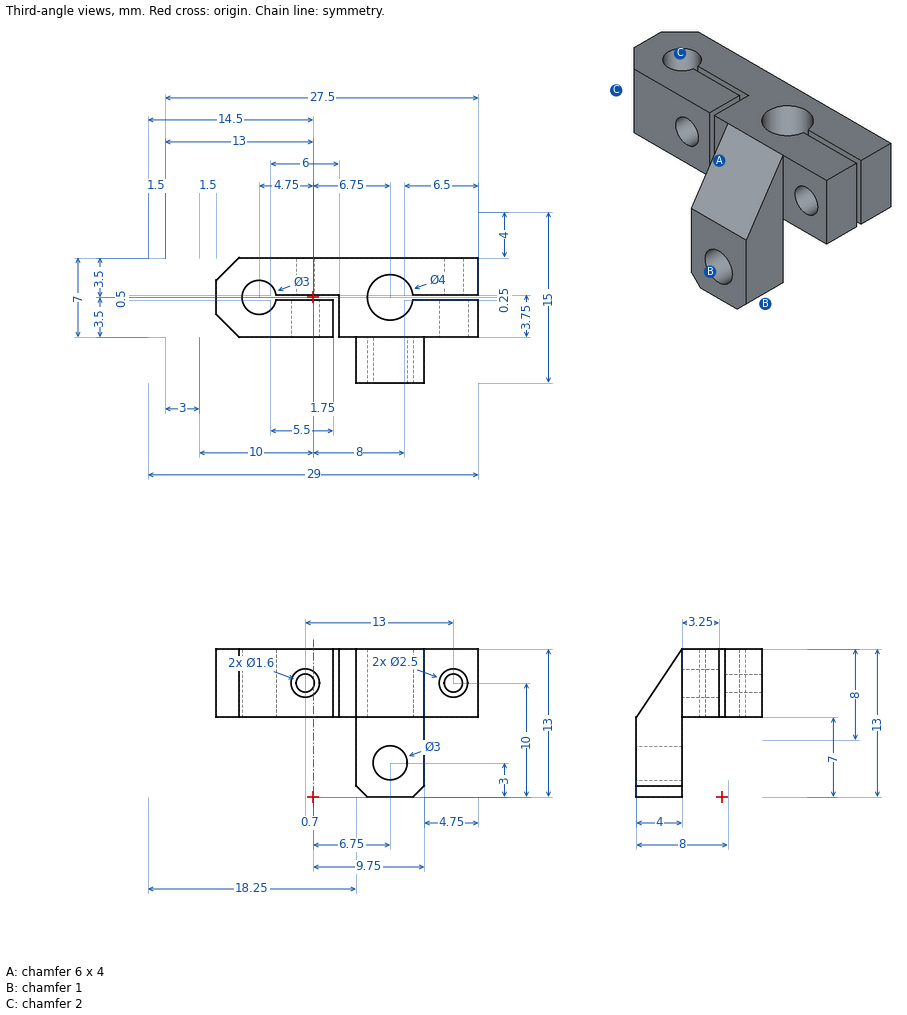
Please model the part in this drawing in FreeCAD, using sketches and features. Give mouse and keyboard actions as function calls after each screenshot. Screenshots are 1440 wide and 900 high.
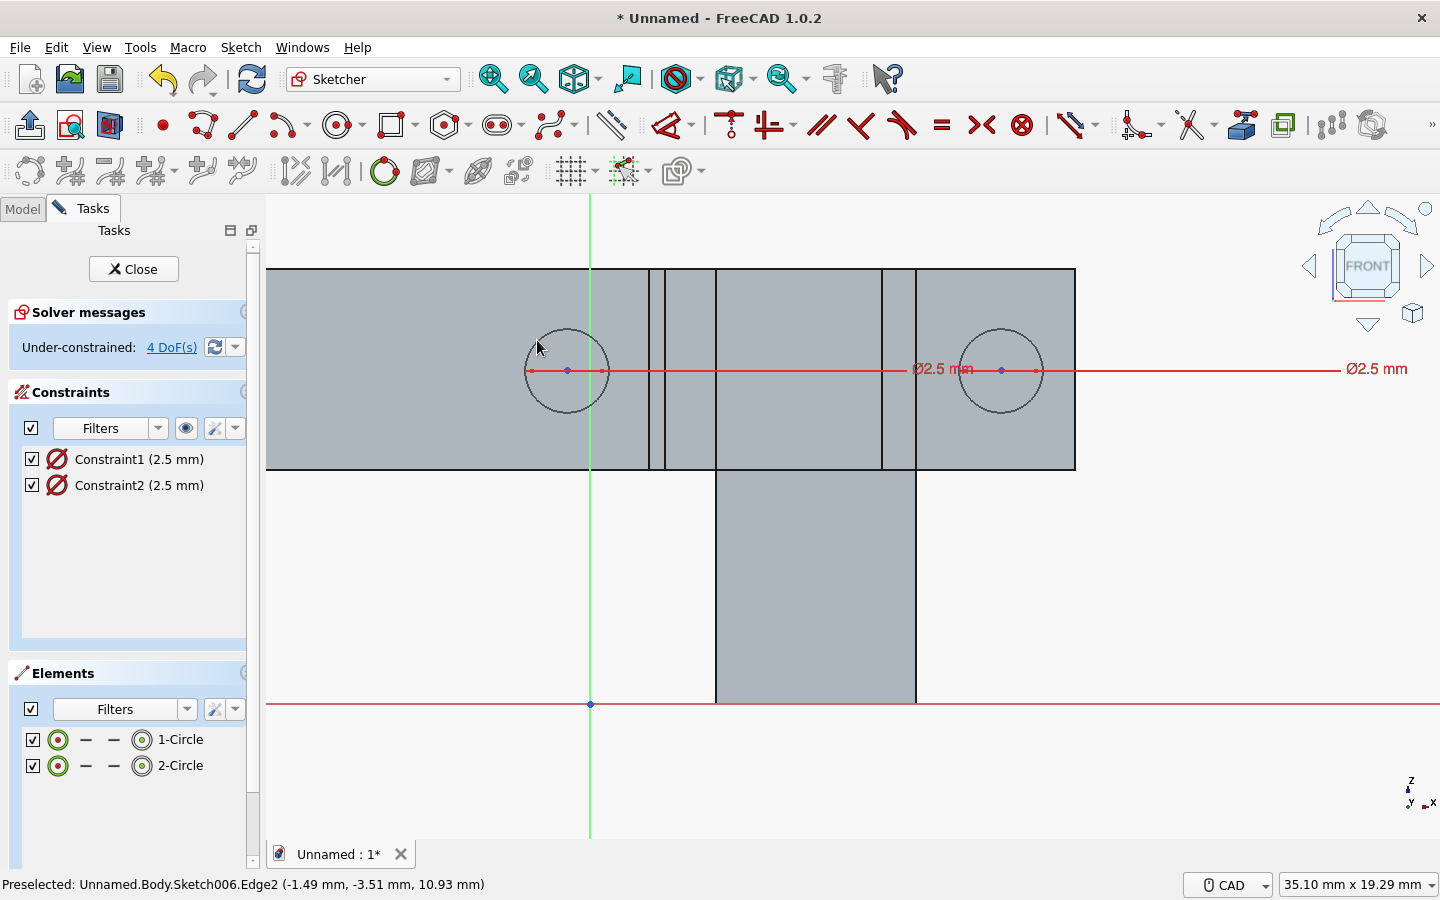
click(1001, 371)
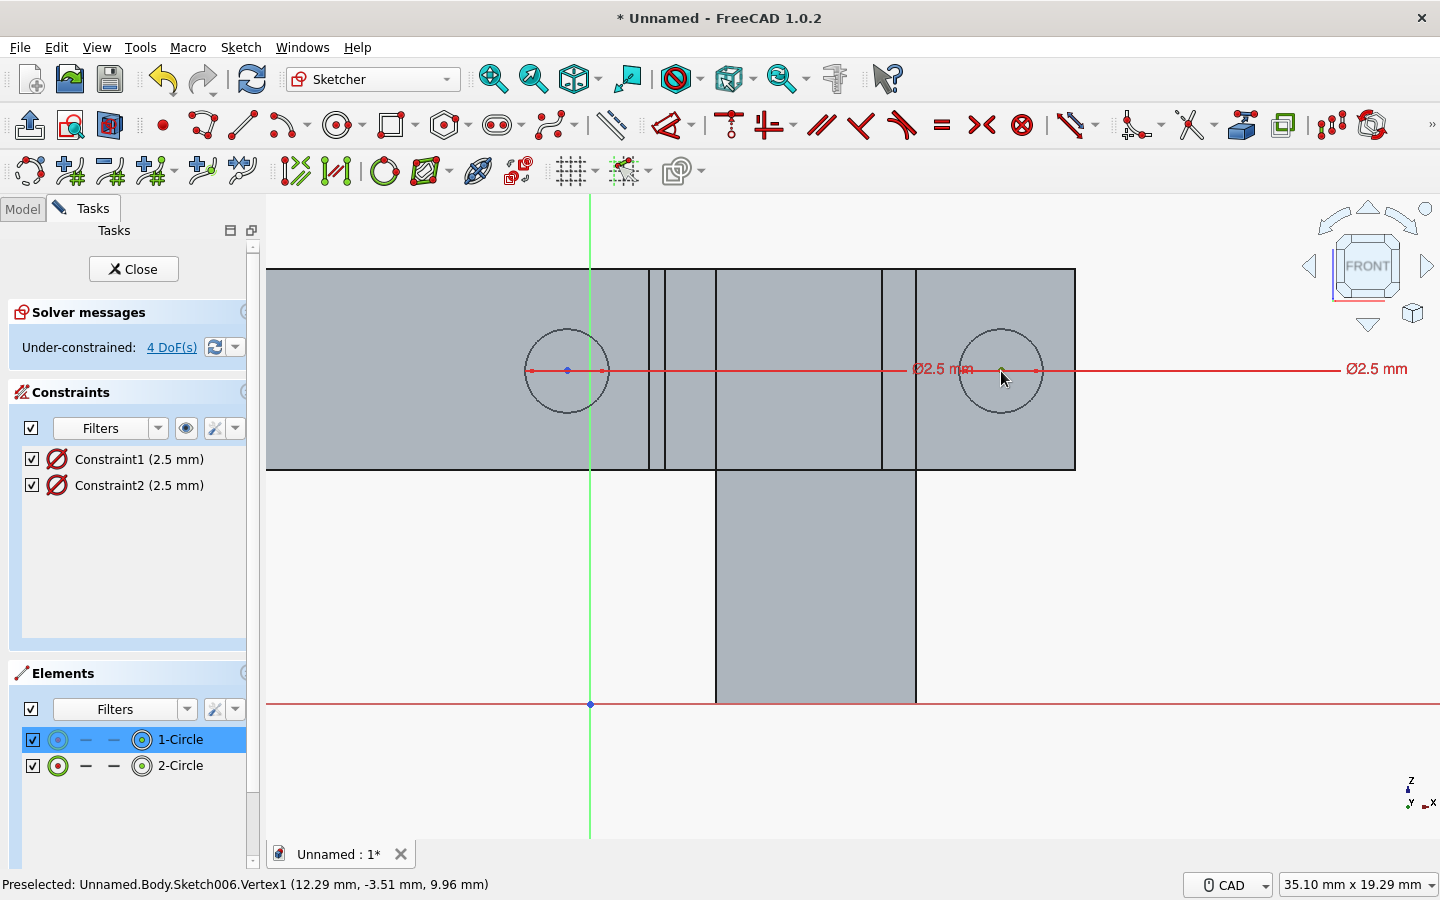
click(567, 371)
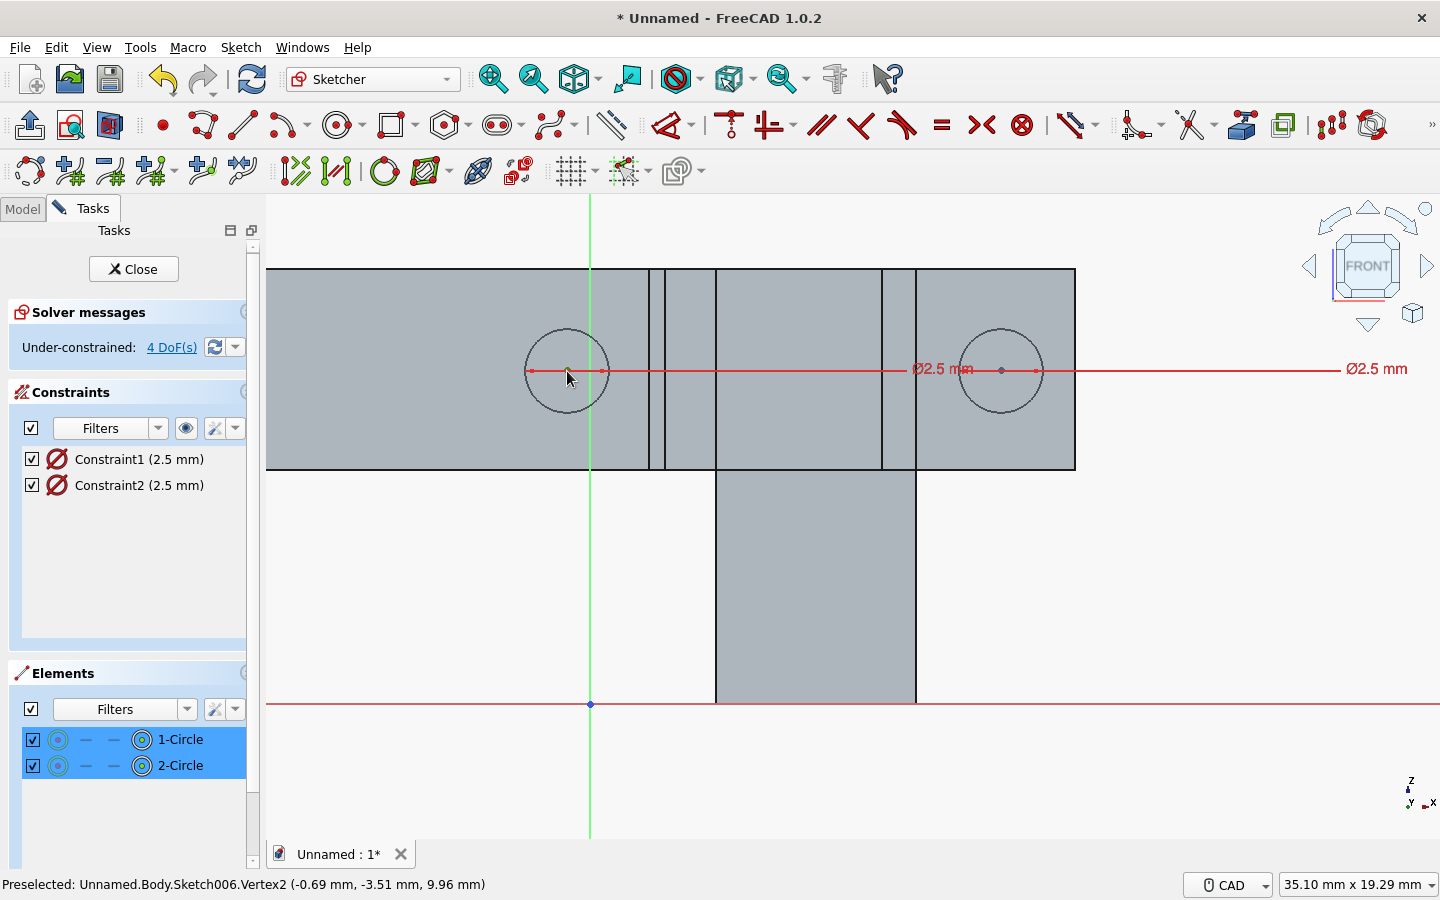
click(796, 126)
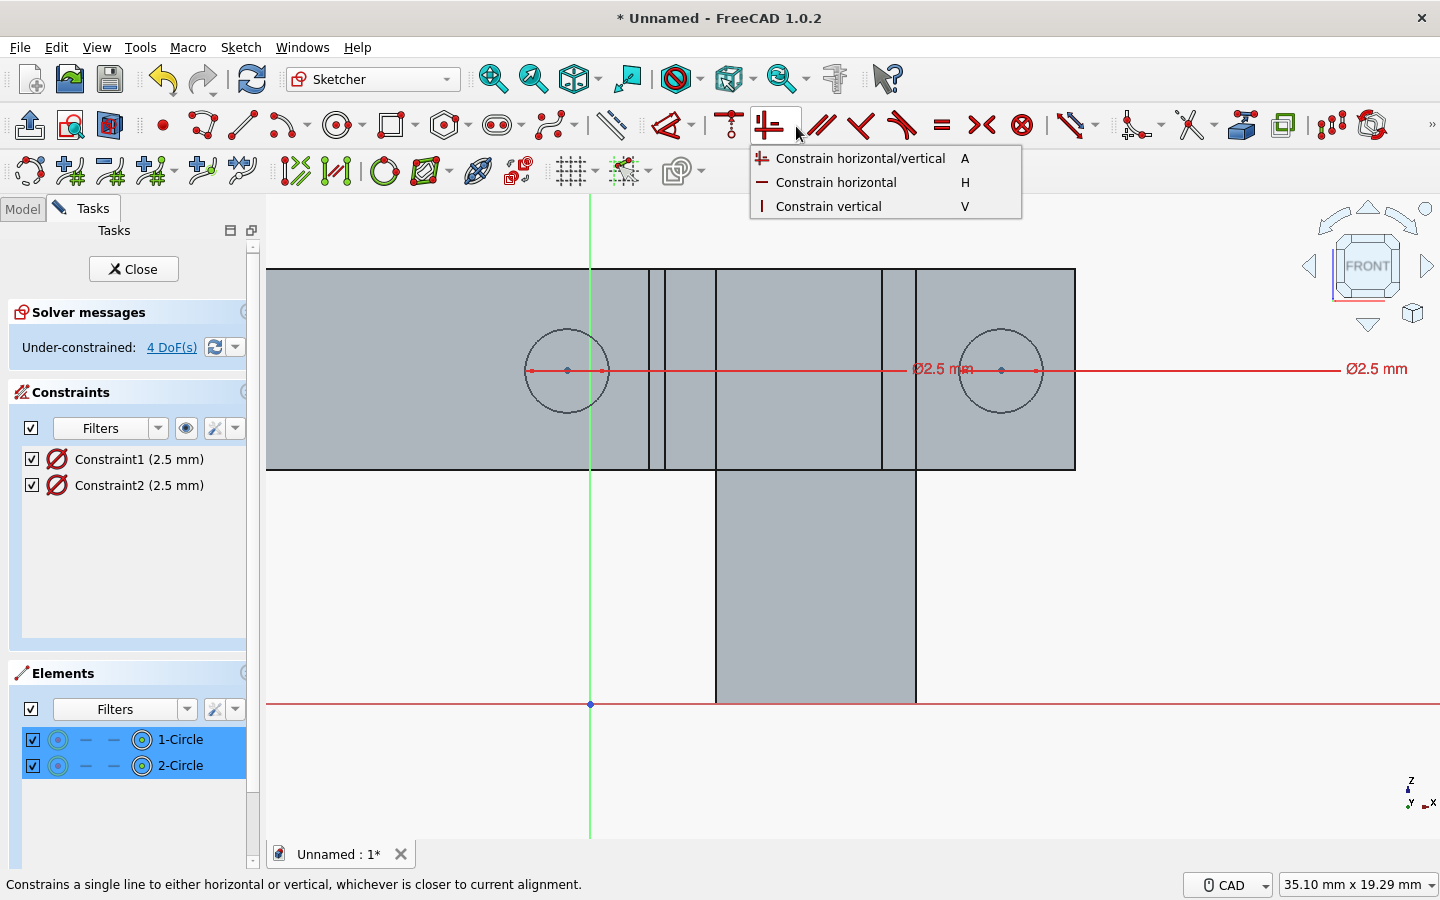
click(886, 182)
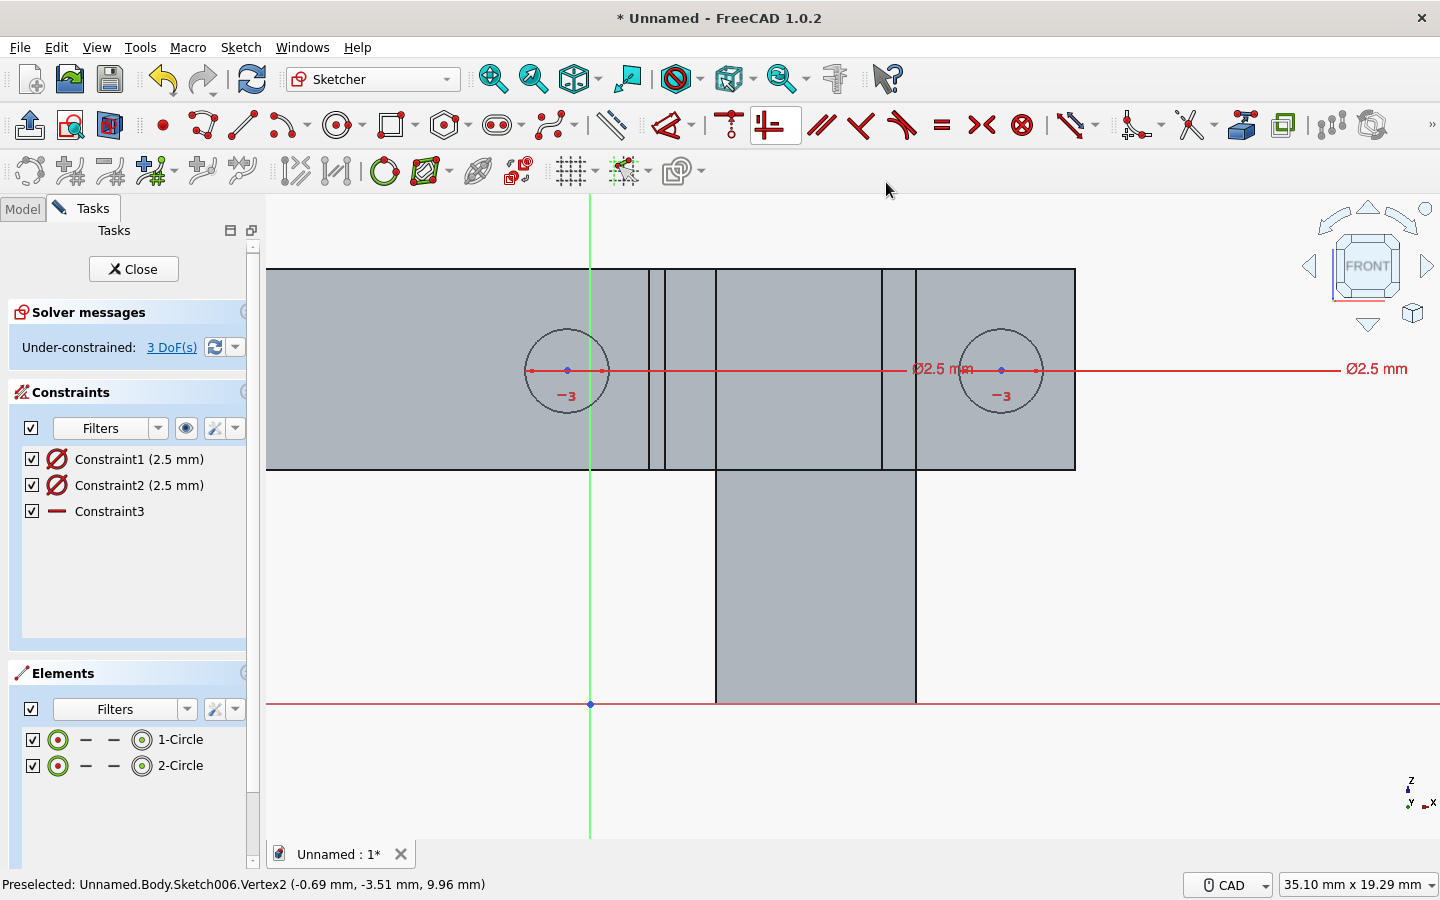
click(666, 126)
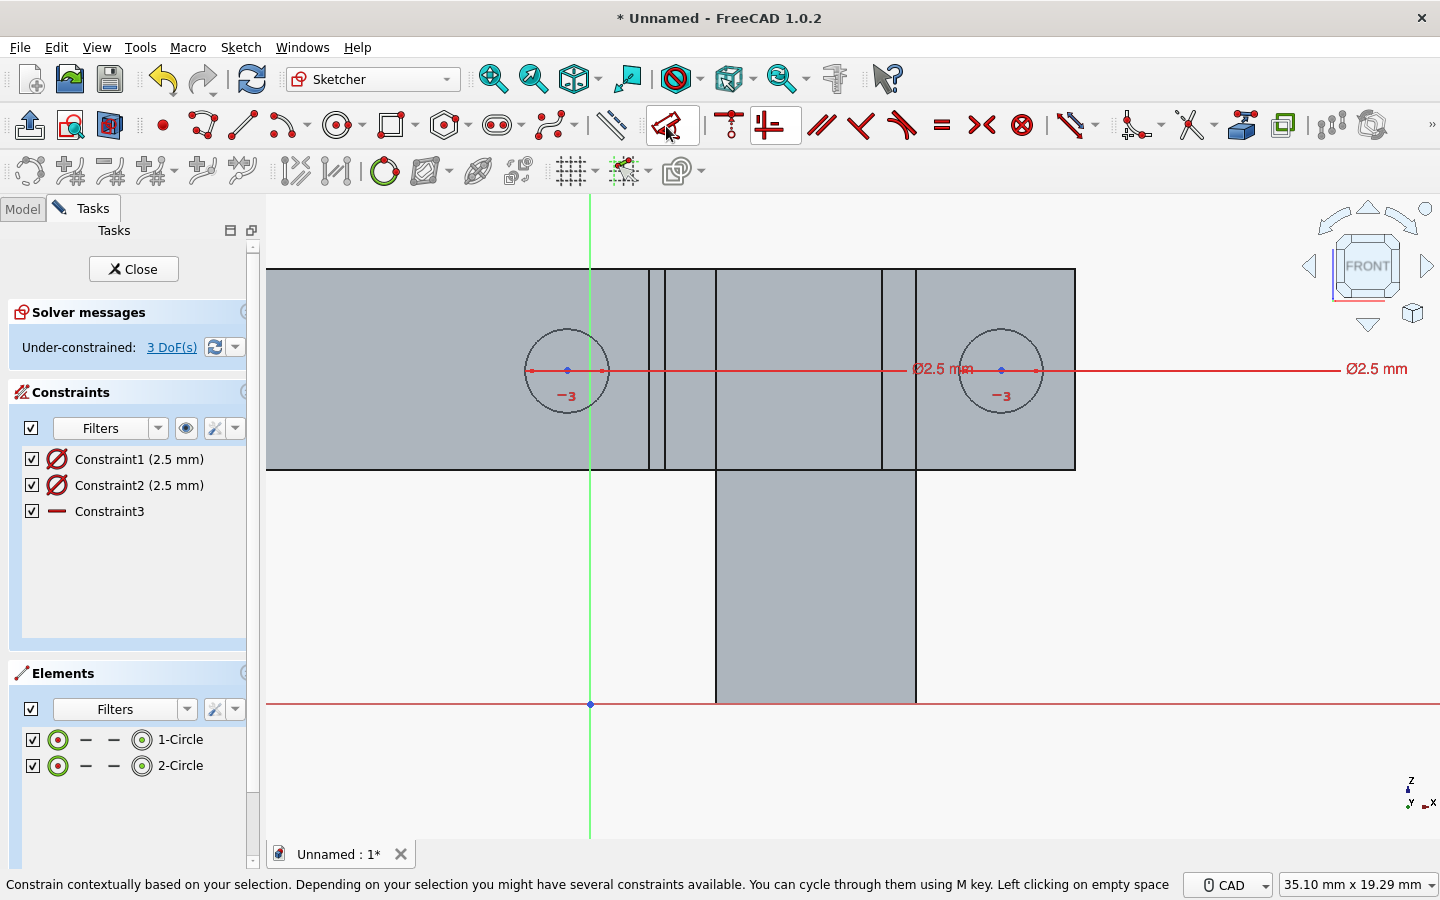
click(1001, 371)
click(1035, 538)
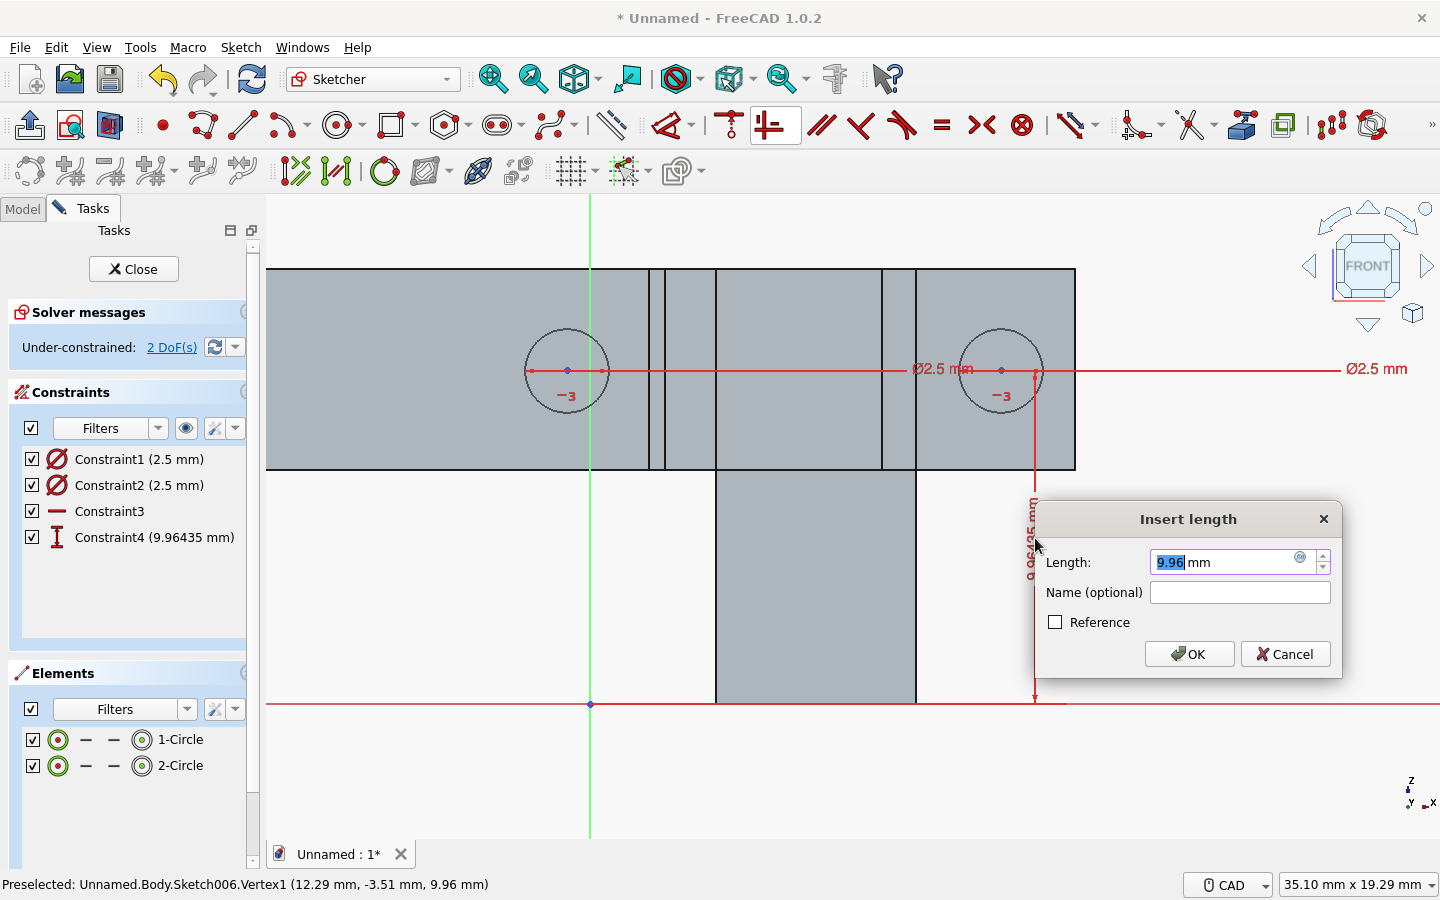
text(10)
key(Return)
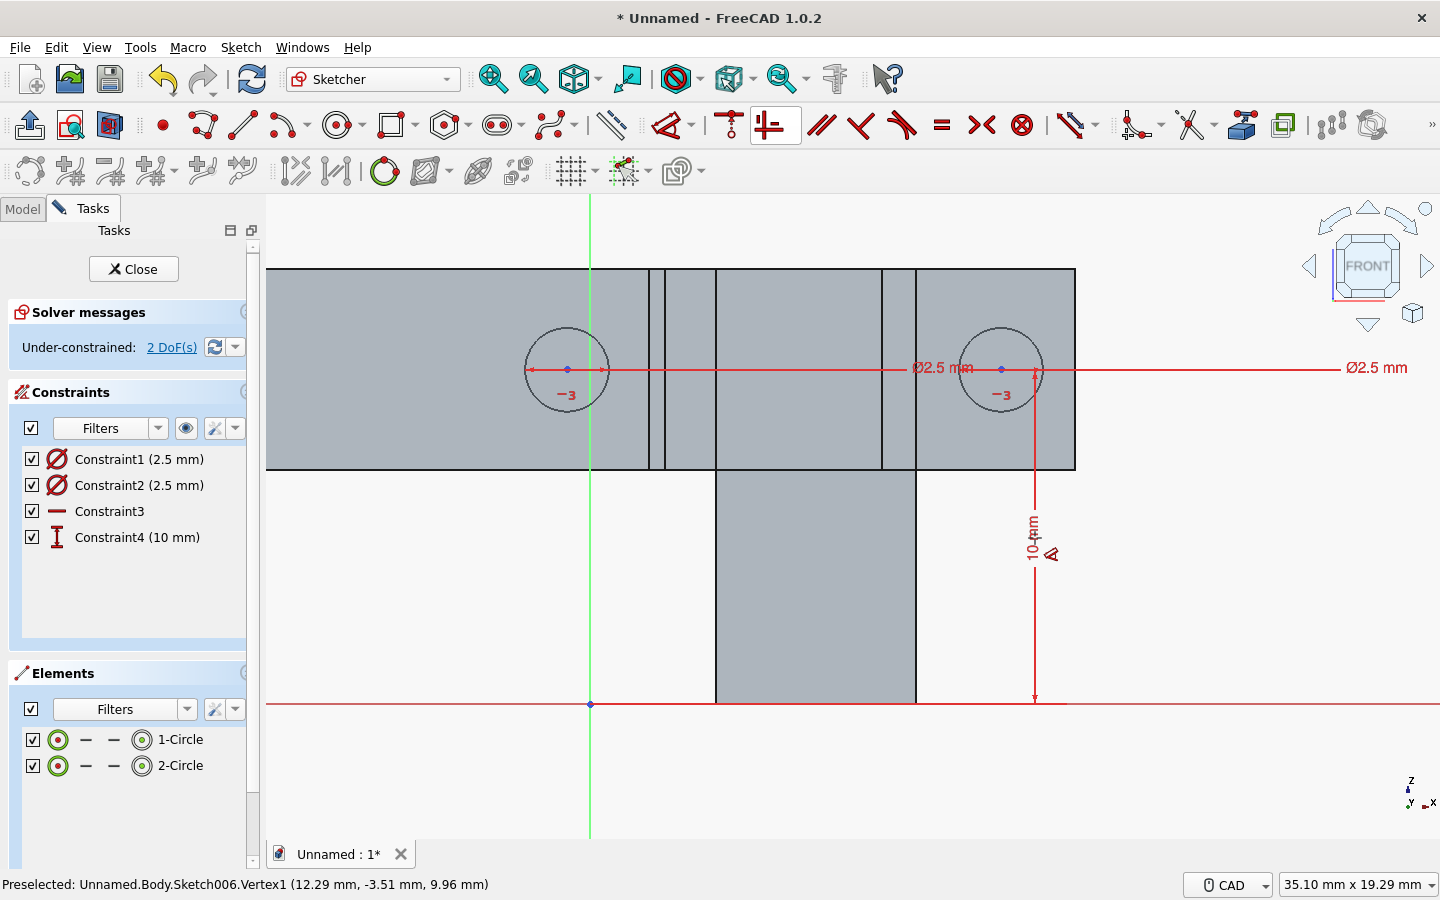
scroll(567, 370, up, 3)